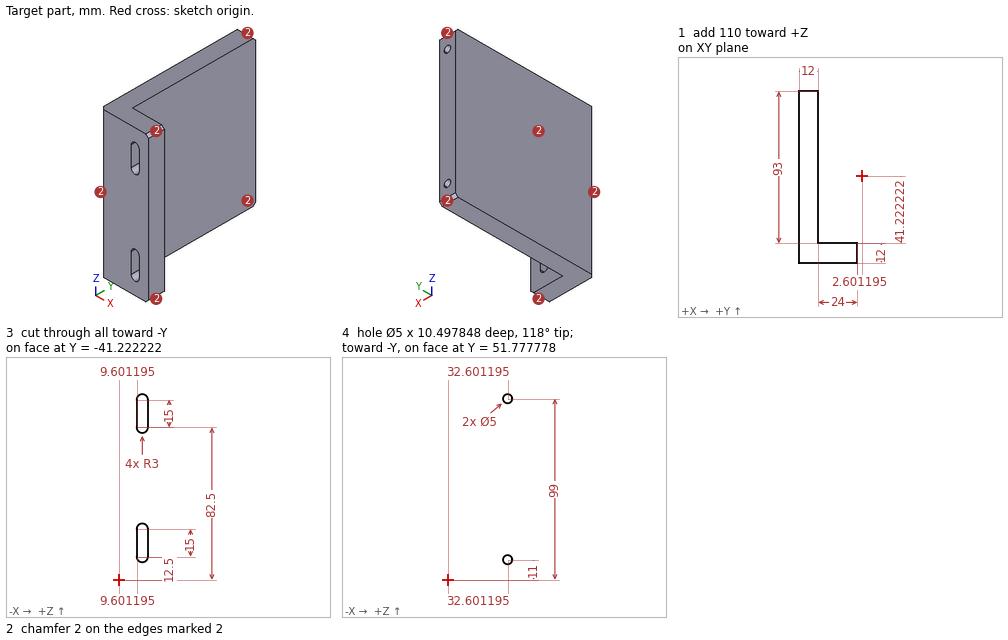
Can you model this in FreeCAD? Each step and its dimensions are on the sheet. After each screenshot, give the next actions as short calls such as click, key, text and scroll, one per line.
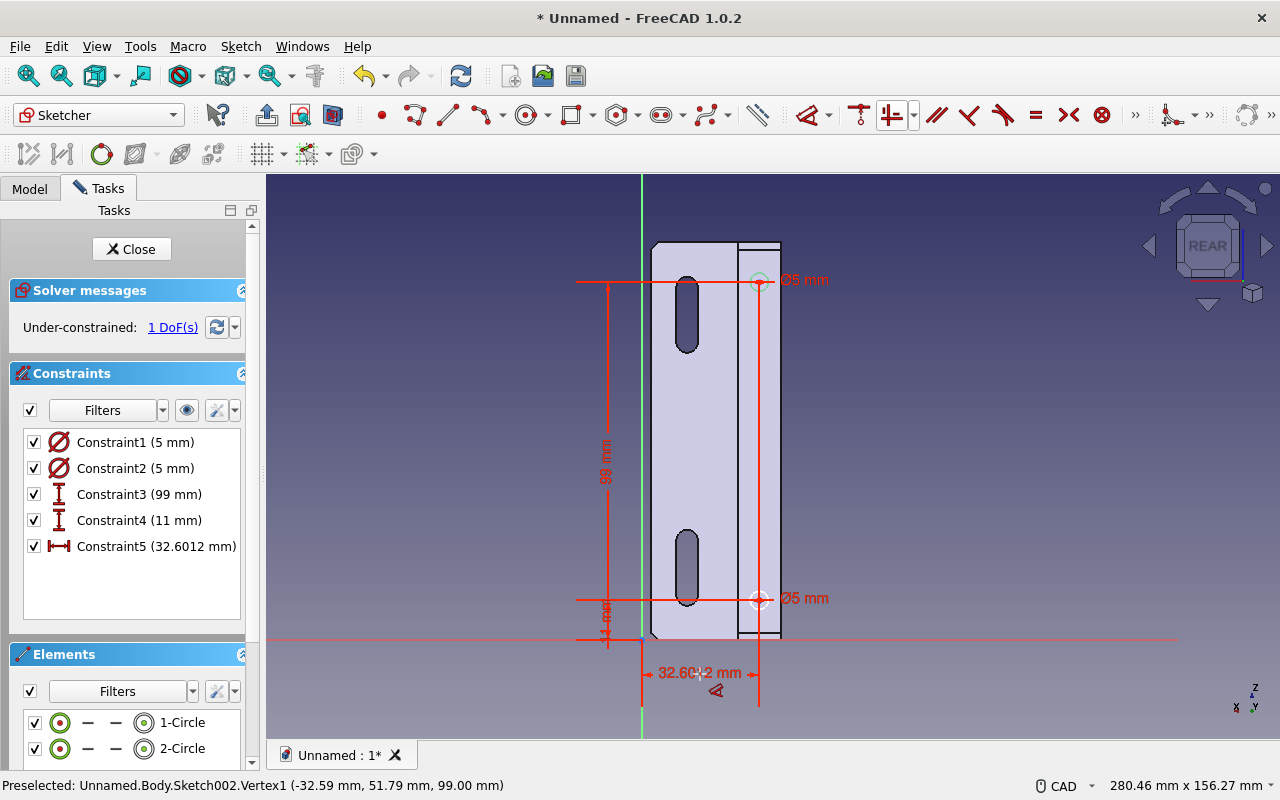
click(759, 600)
click(700, 566)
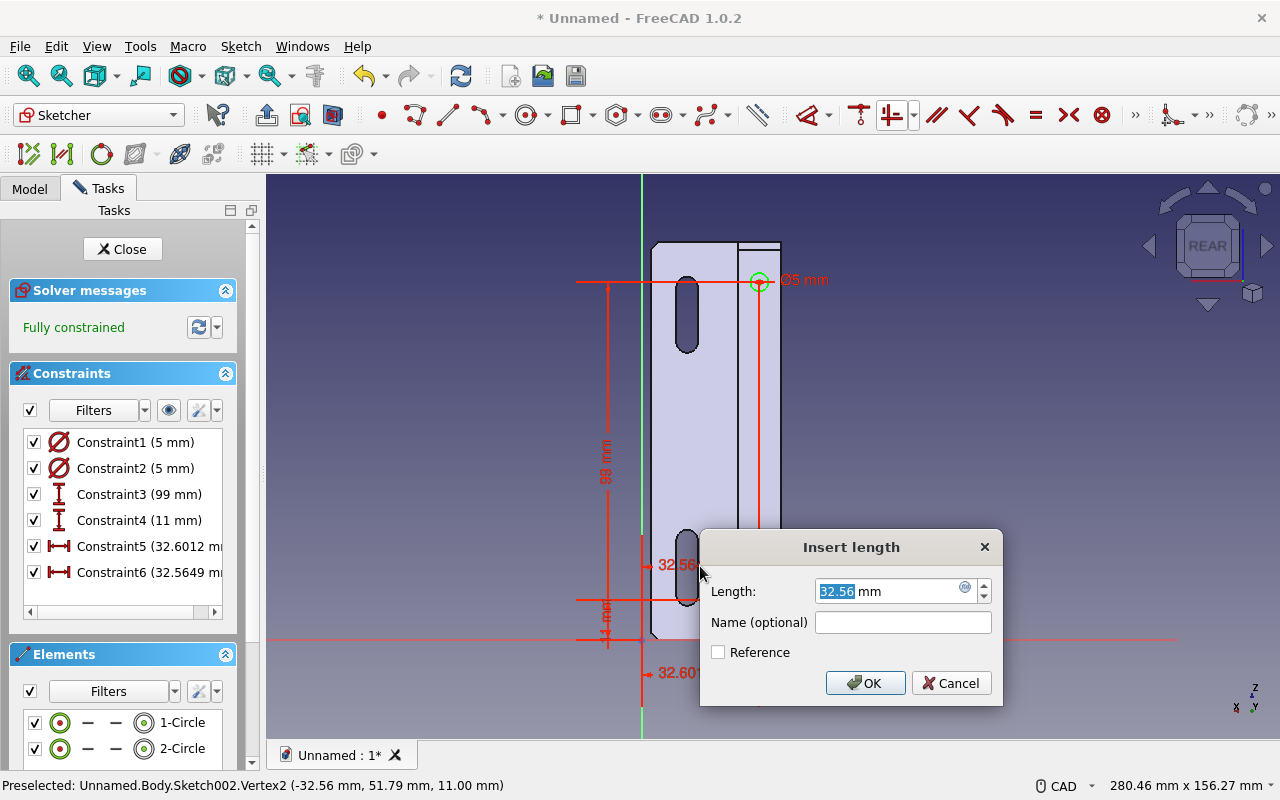
text(32.601195)
key(Return)
key(Escape)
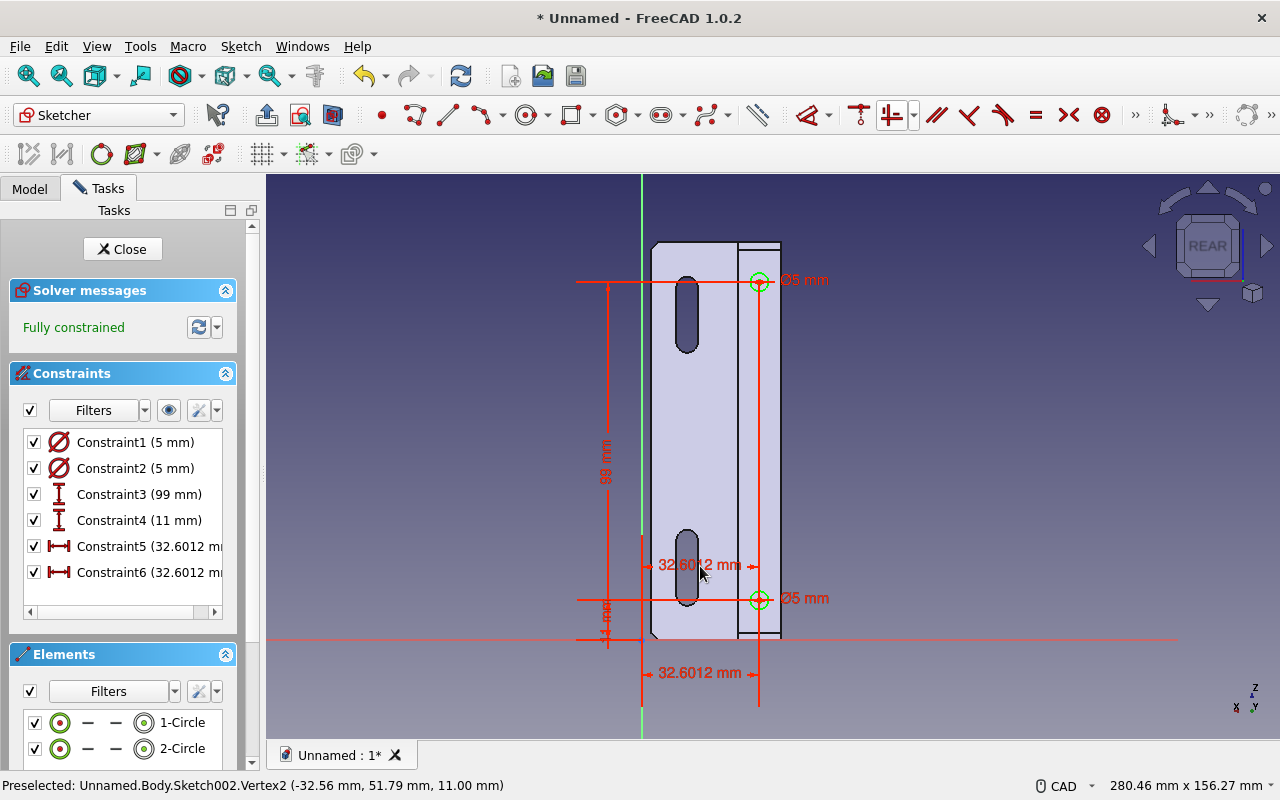
click(123, 249)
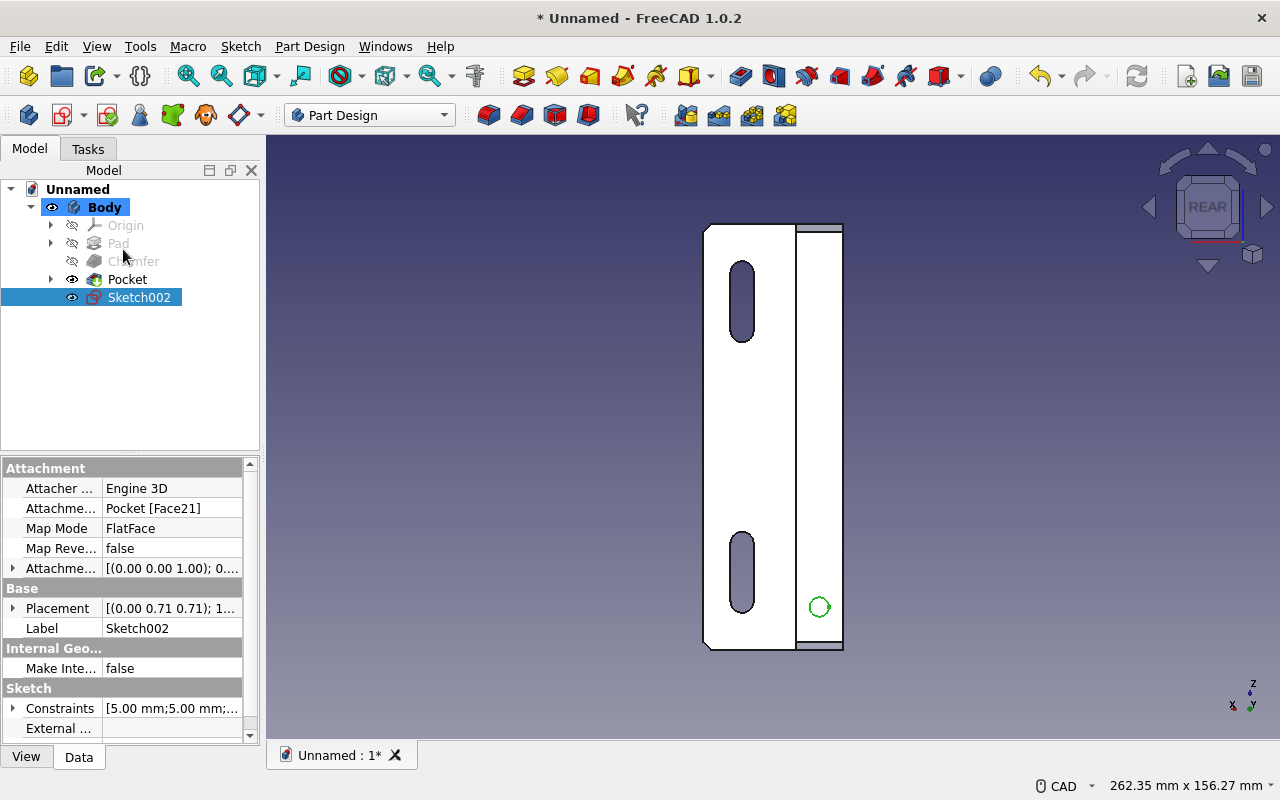
click(774, 76)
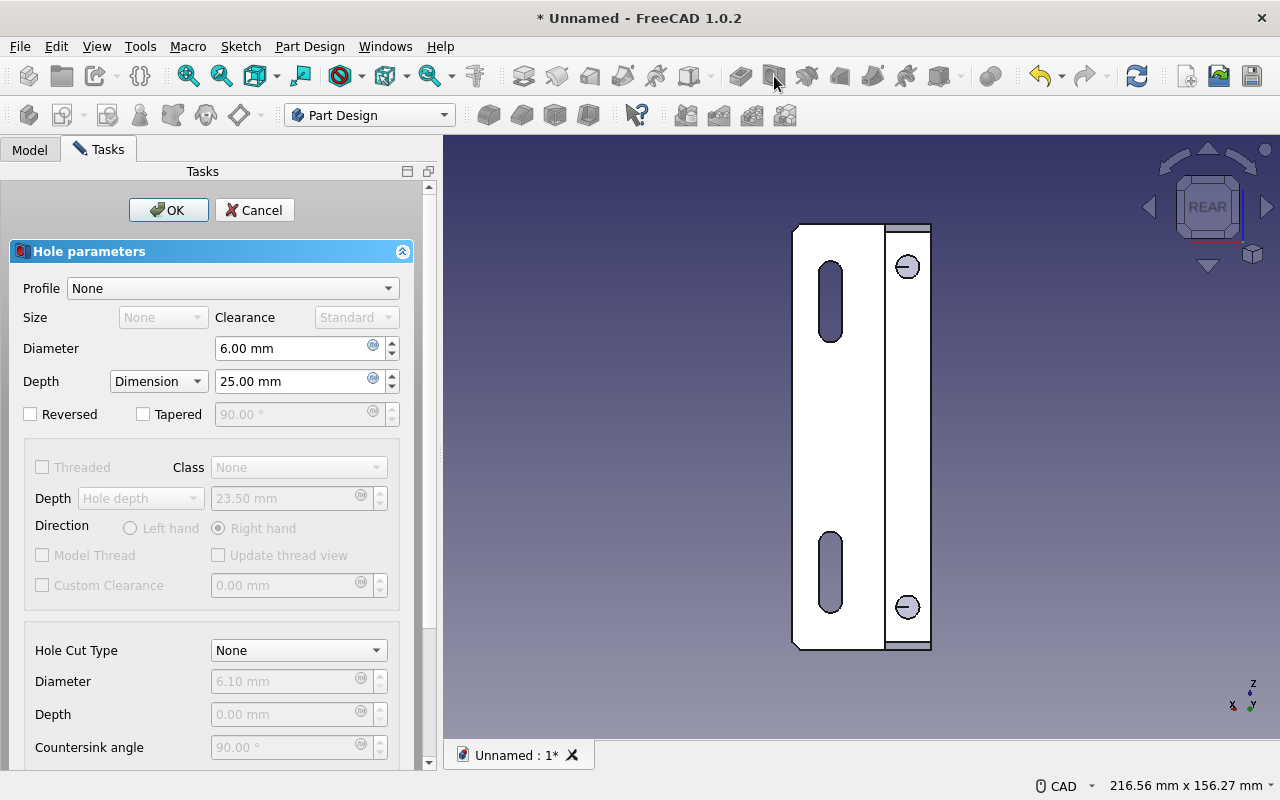
triple_click(300, 348)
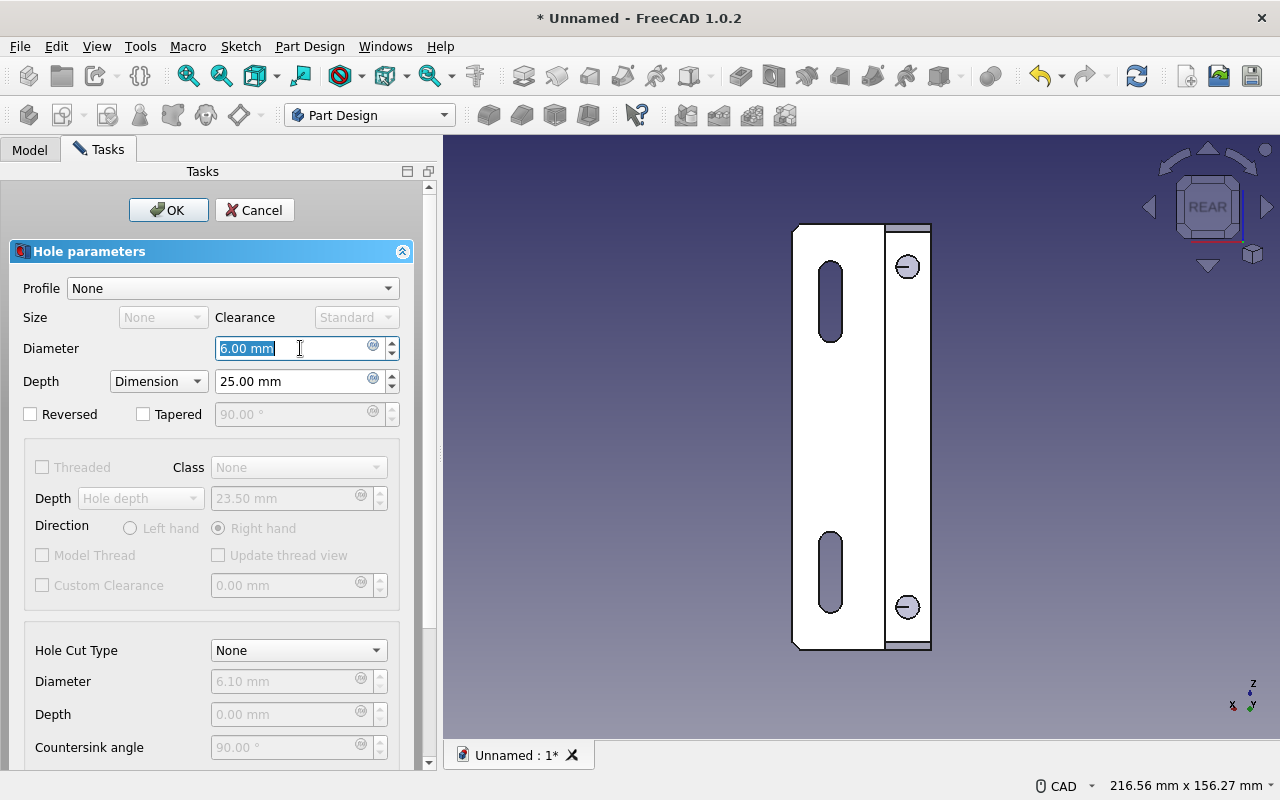
text(5)
key(Tab)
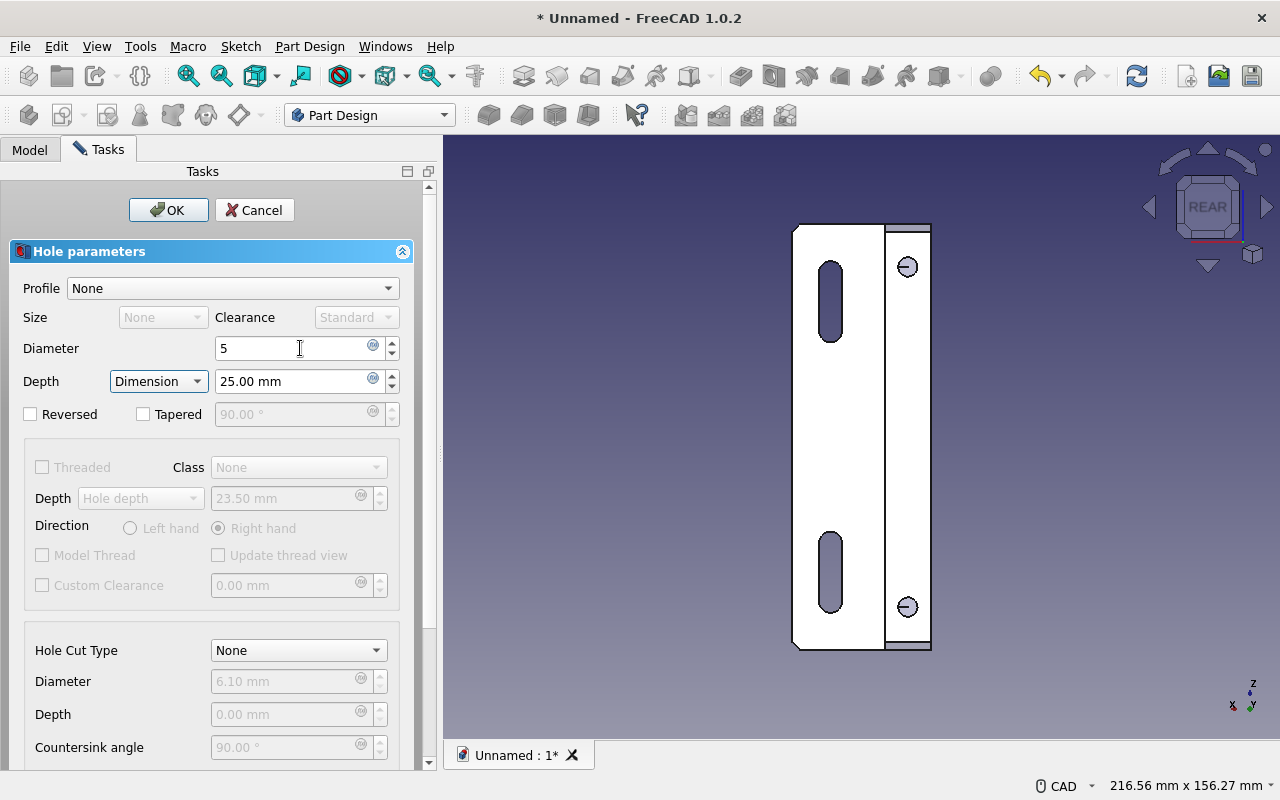
triple_click(300, 382)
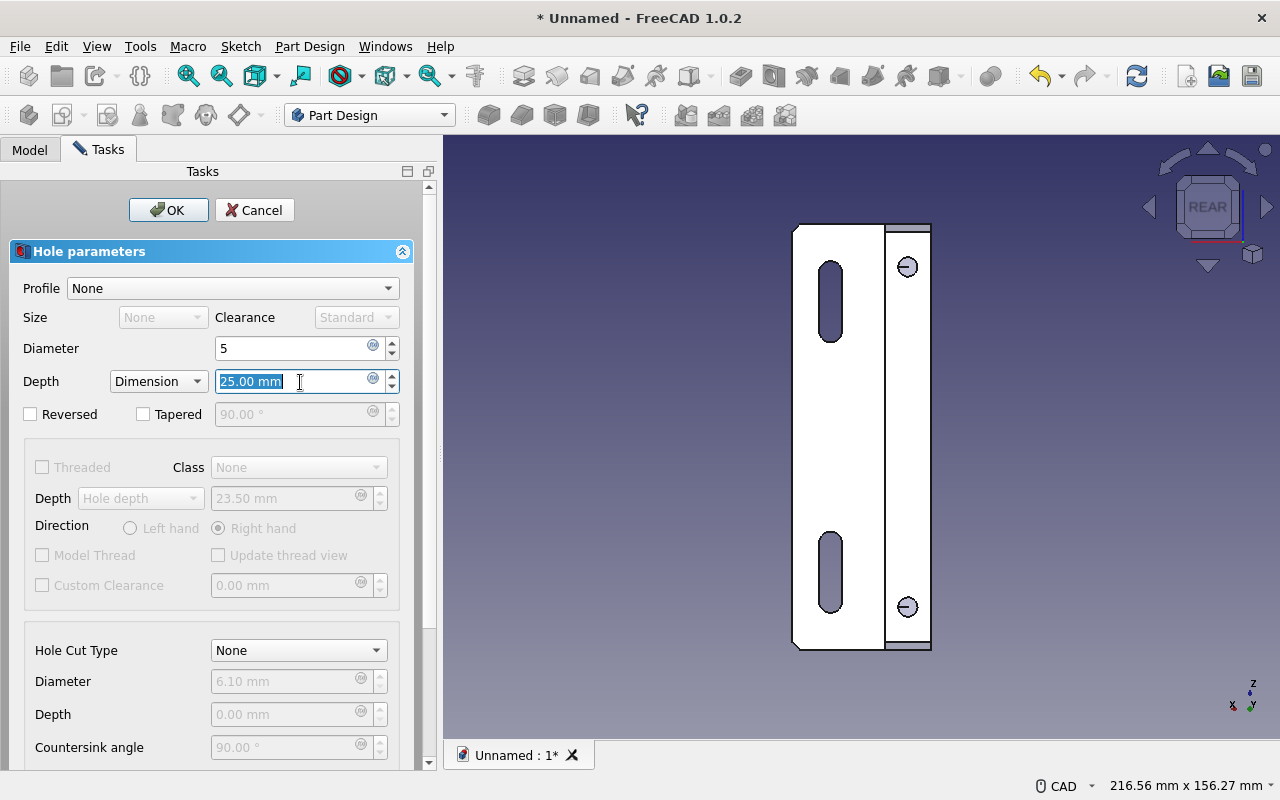
text(10.497848)
key(Tab)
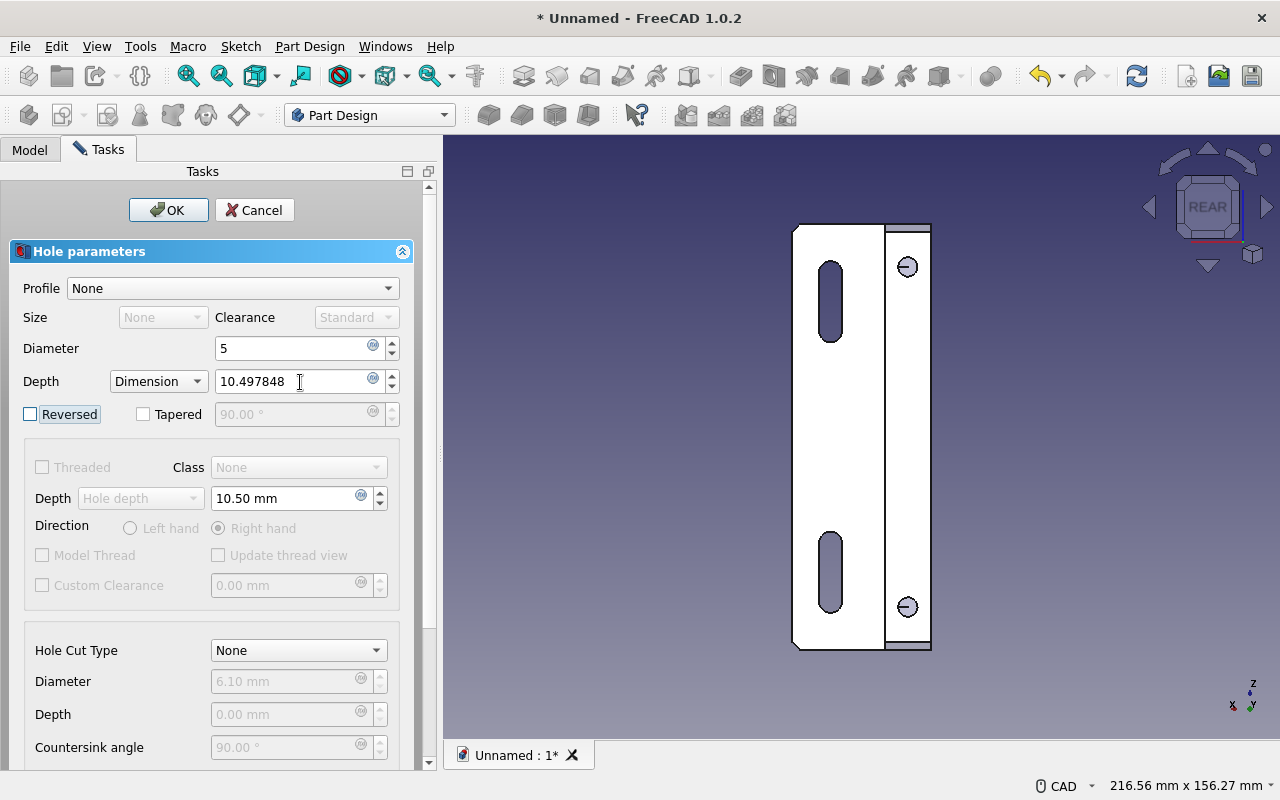
click(169, 210)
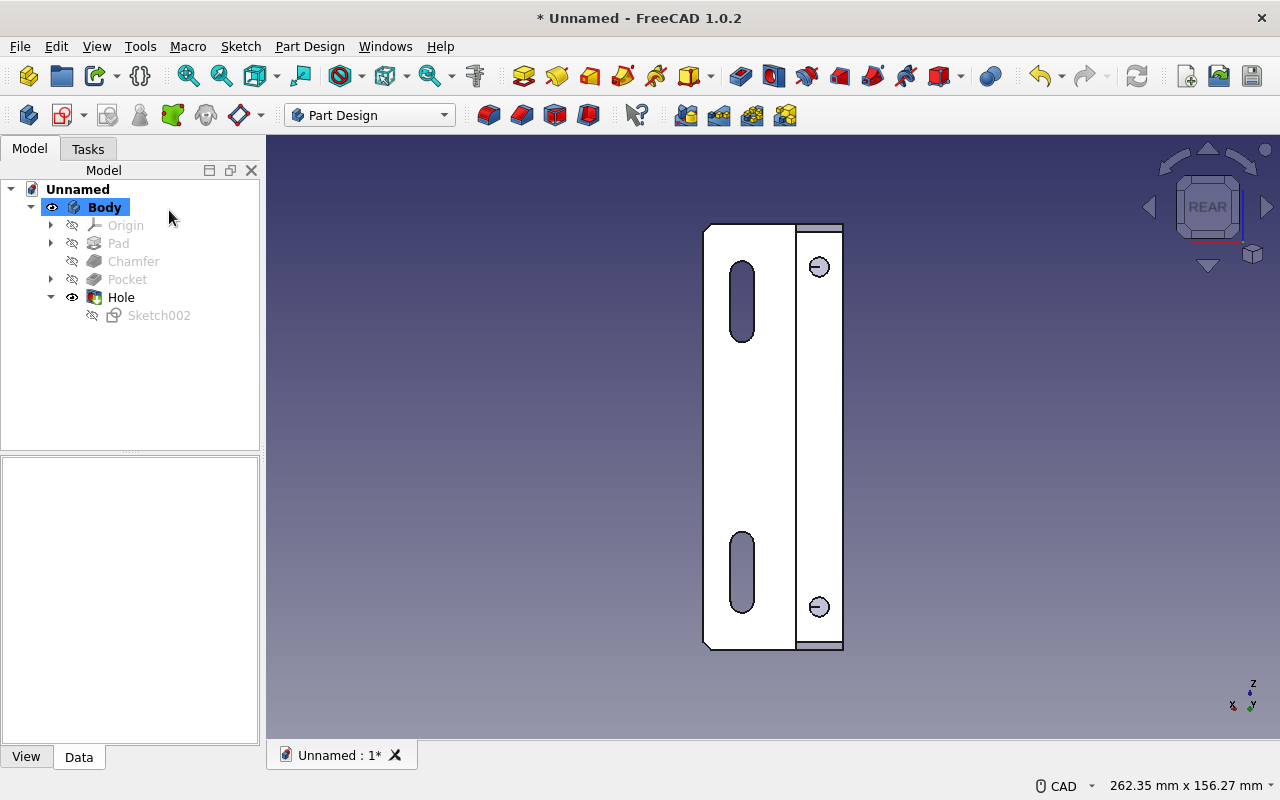
key(0)